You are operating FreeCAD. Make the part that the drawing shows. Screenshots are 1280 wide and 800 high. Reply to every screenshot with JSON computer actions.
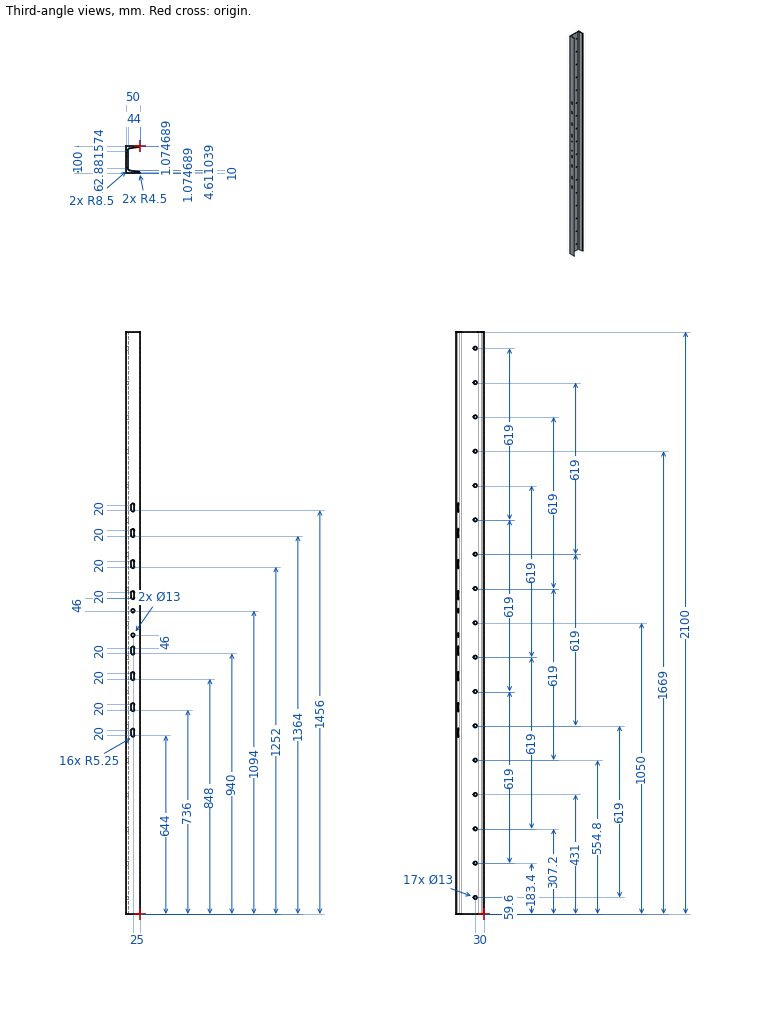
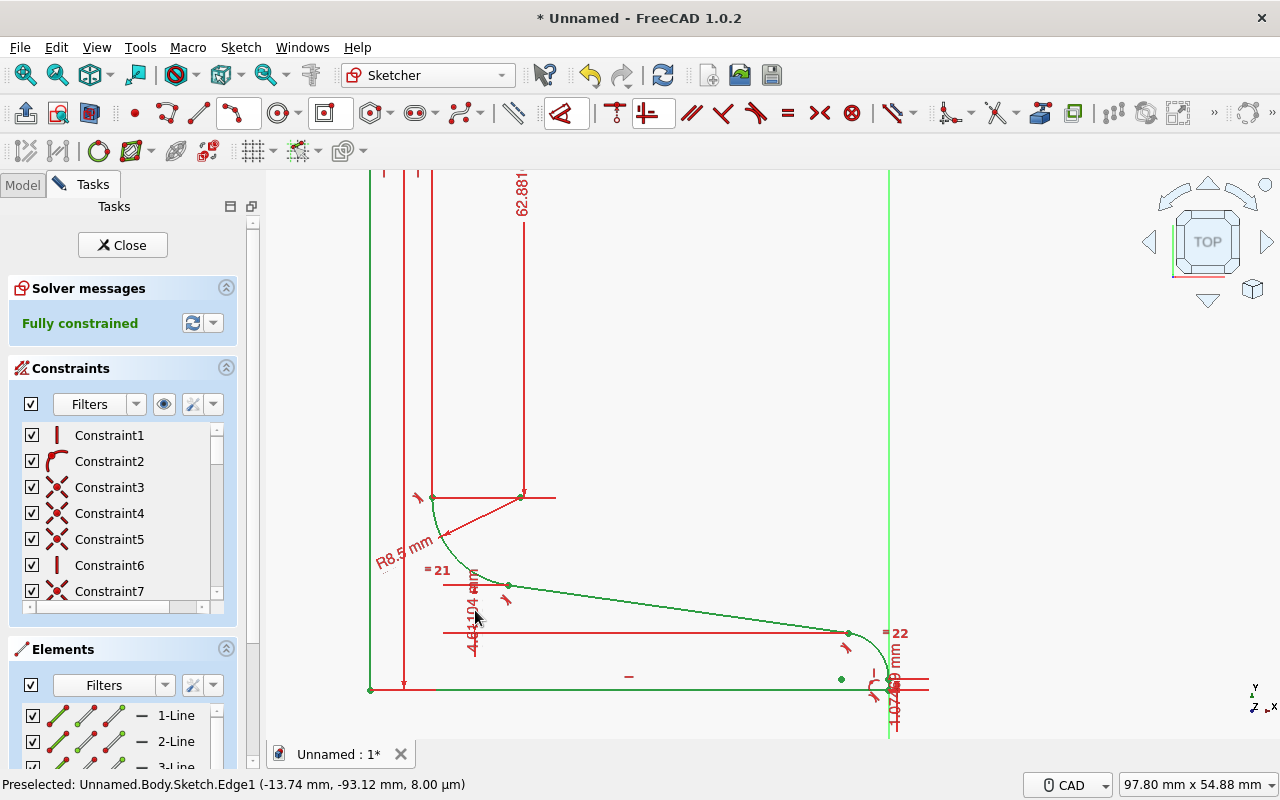
{"action": "left_click", "coordinate": [123, 245]}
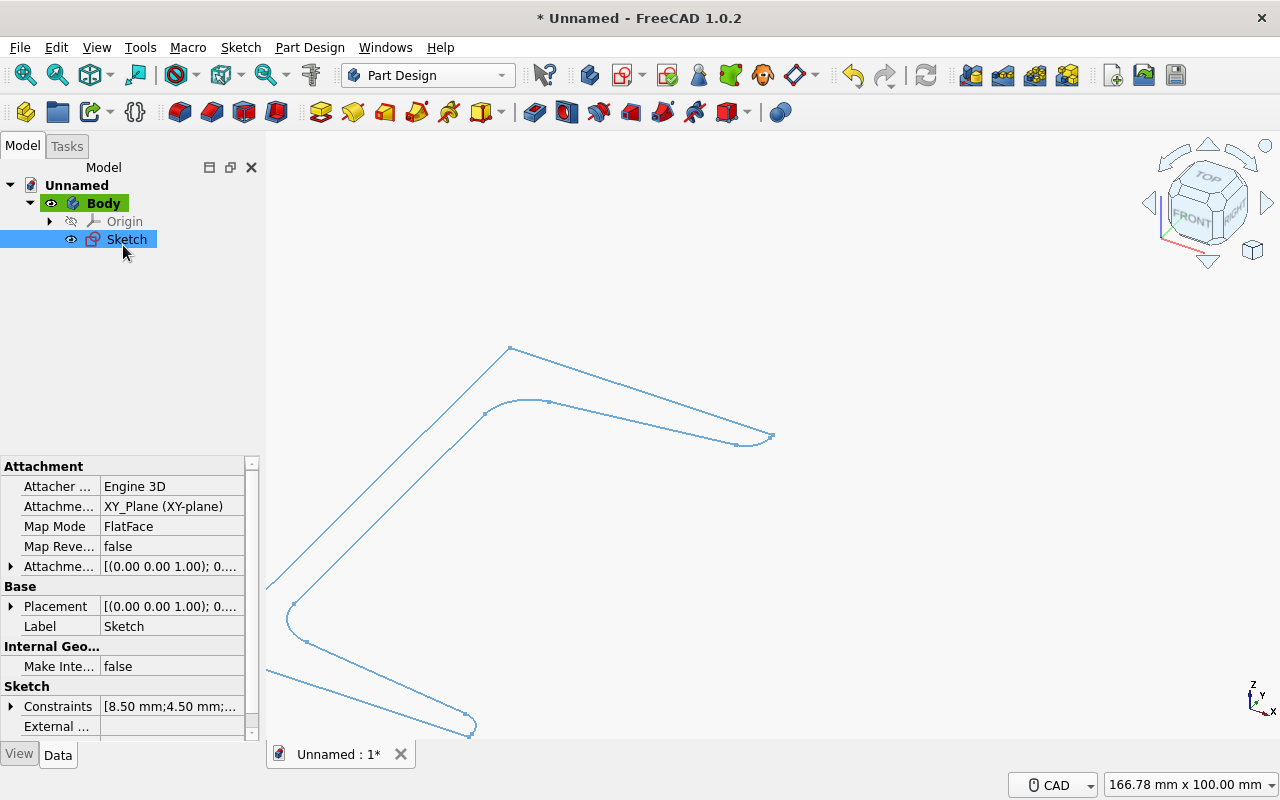
{"action": "left_click", "coordinate": [322, 112]}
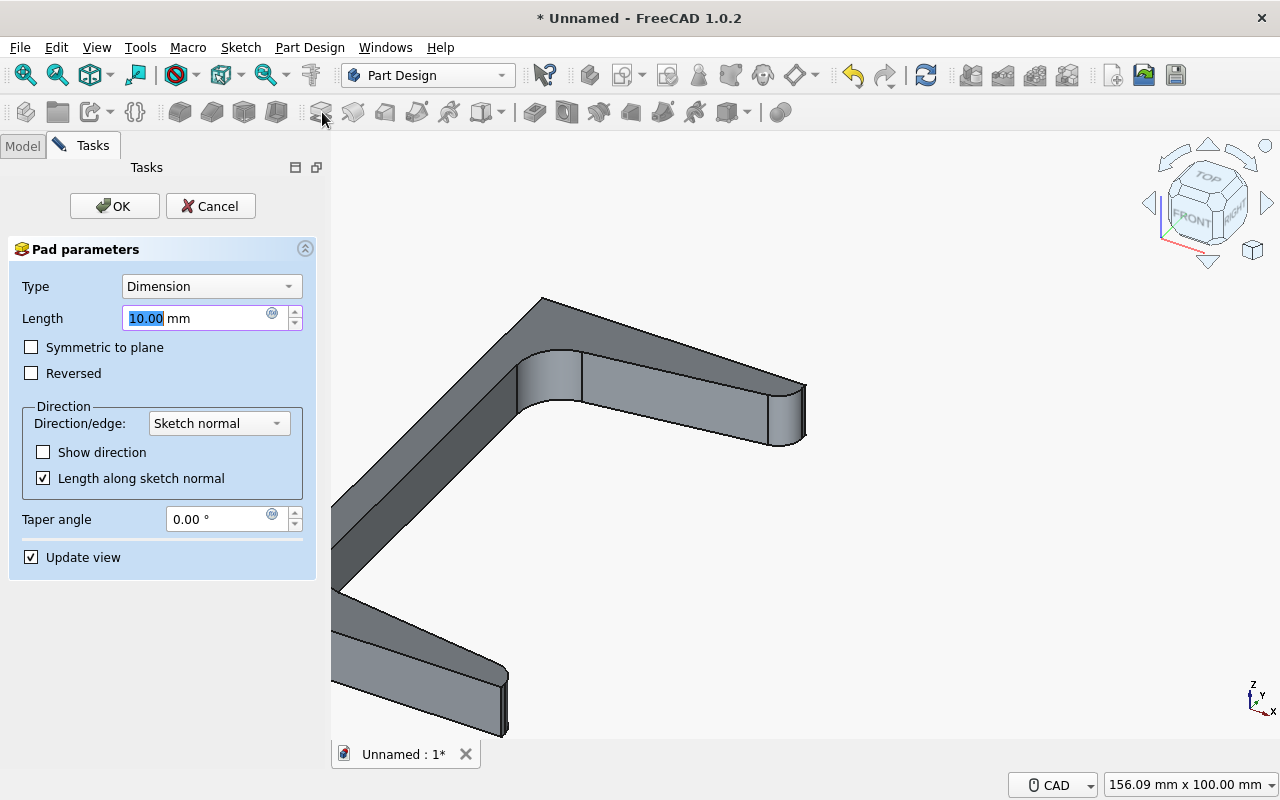
{"action": "type", "text": "2100"}
{"action": "key", "text": "Tab"}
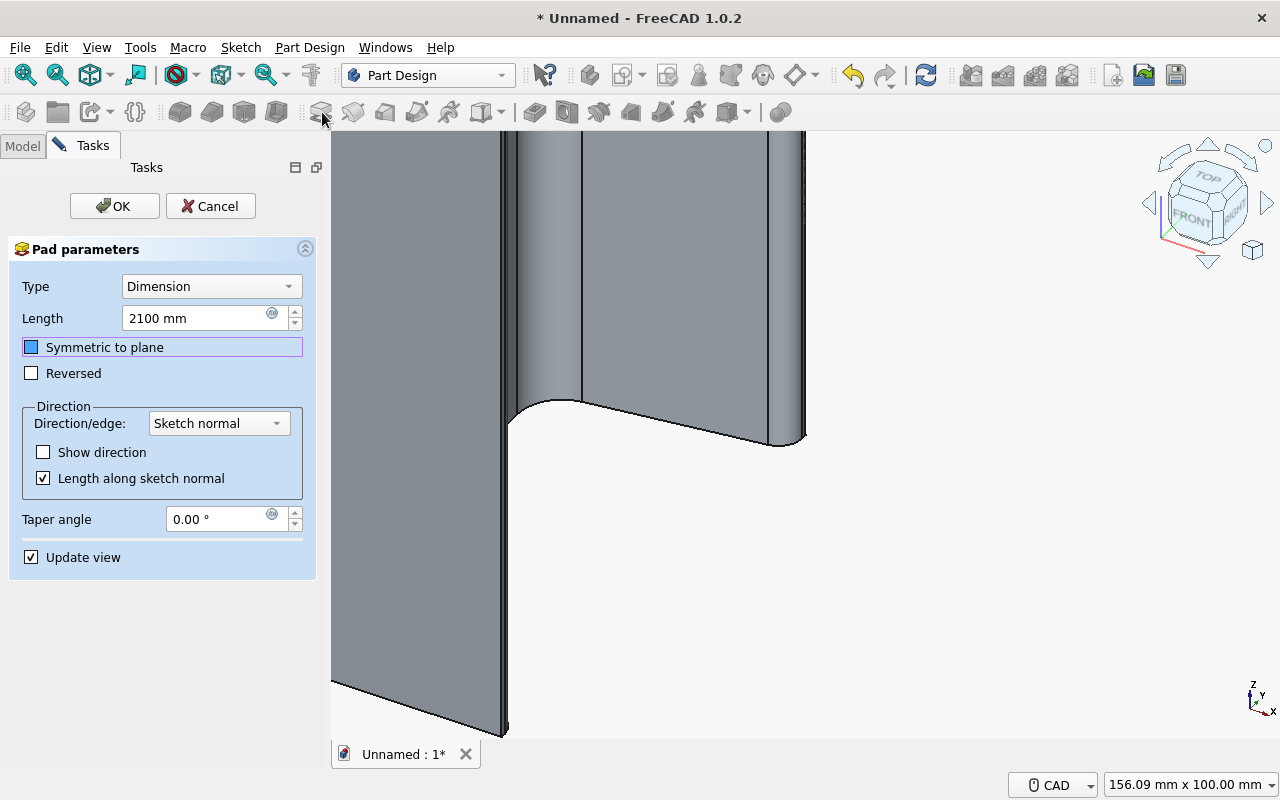
{"action": "left_click", "coordinate": [115, 206]}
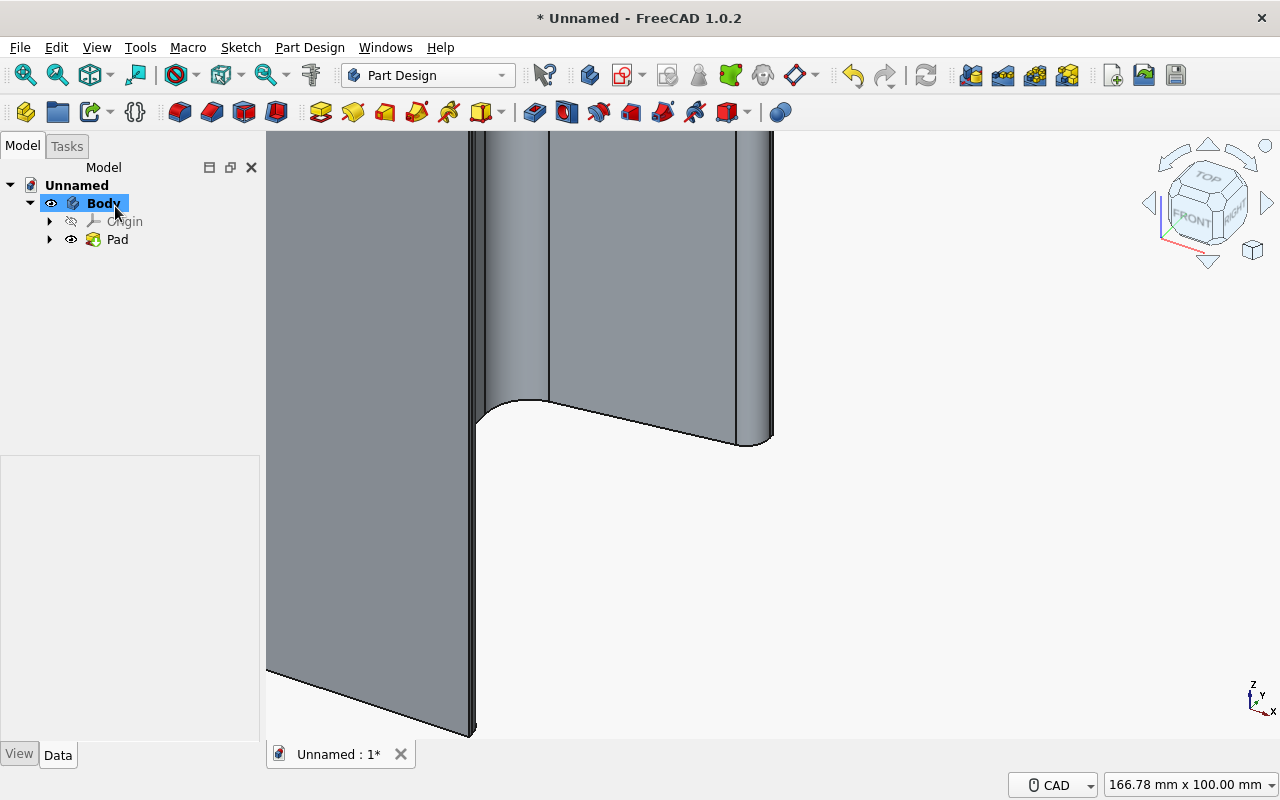
{"action": "left_click", "coordinate": [26, 76]}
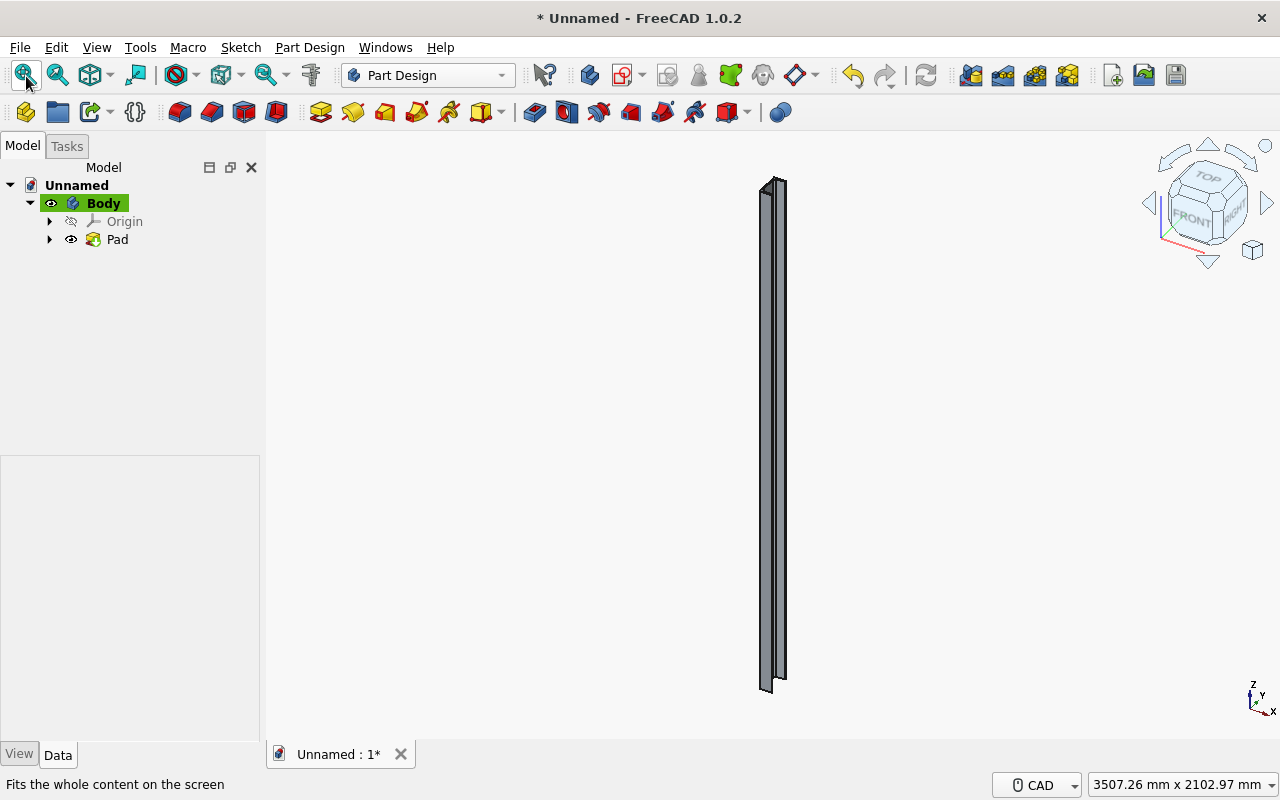
{"action": "key", "text": "6"}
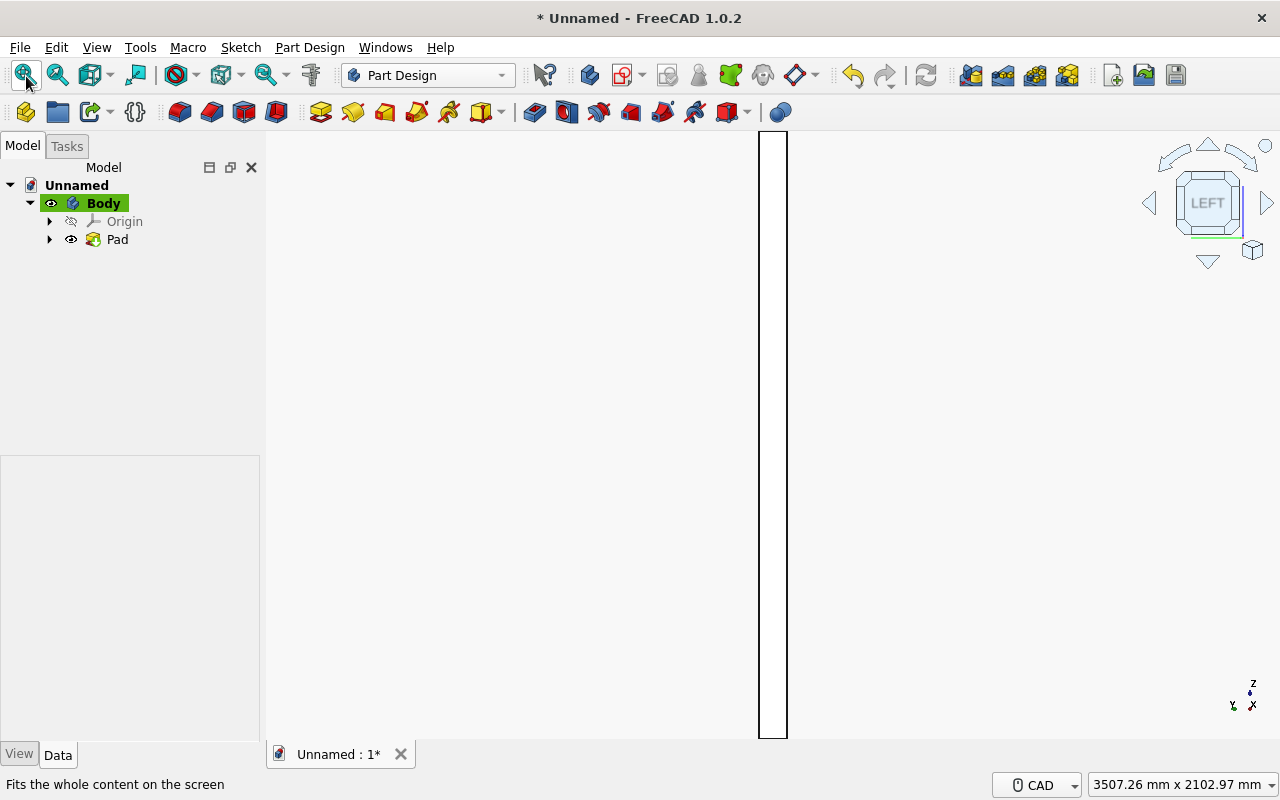
{"action": "left_click", "coordinate": [26, 76]}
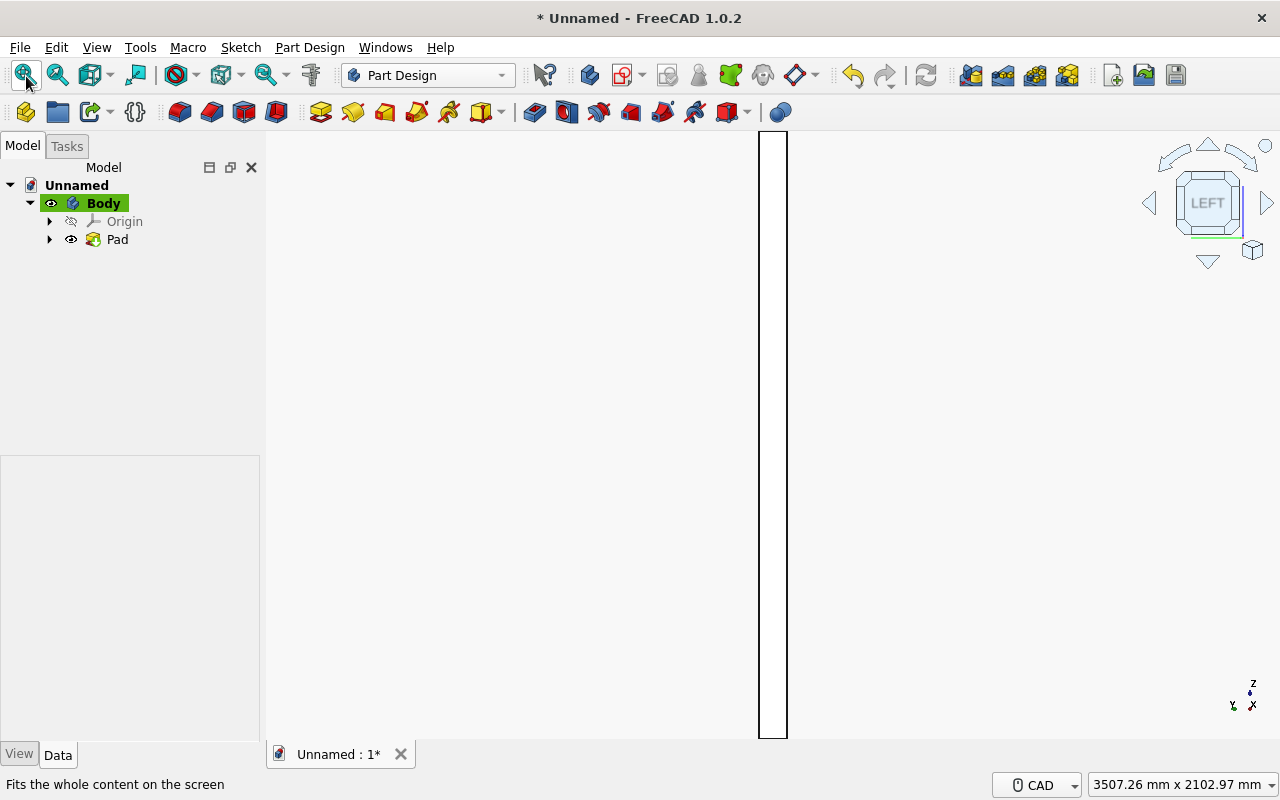
{"action": "left_click", "coordinate": [773, 174]}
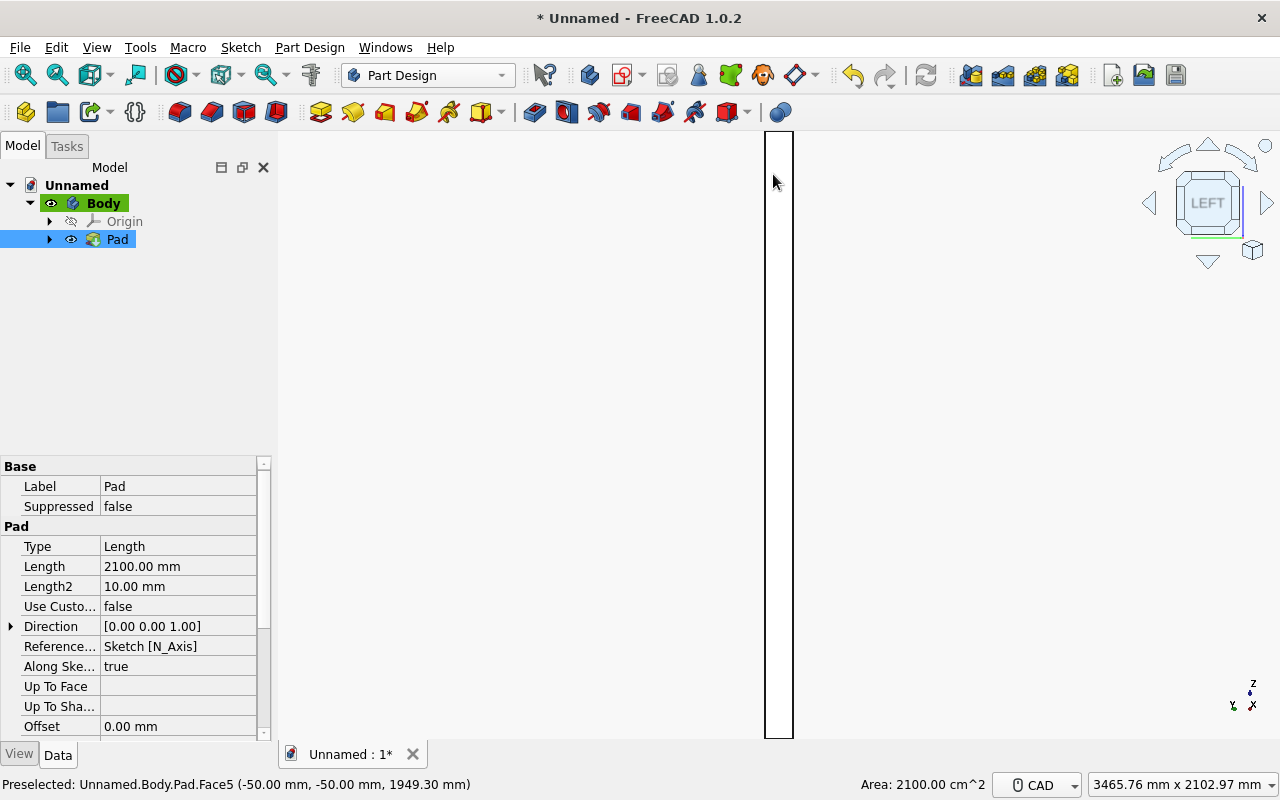
{"action": "left_click", "coordinate": [622, 76]}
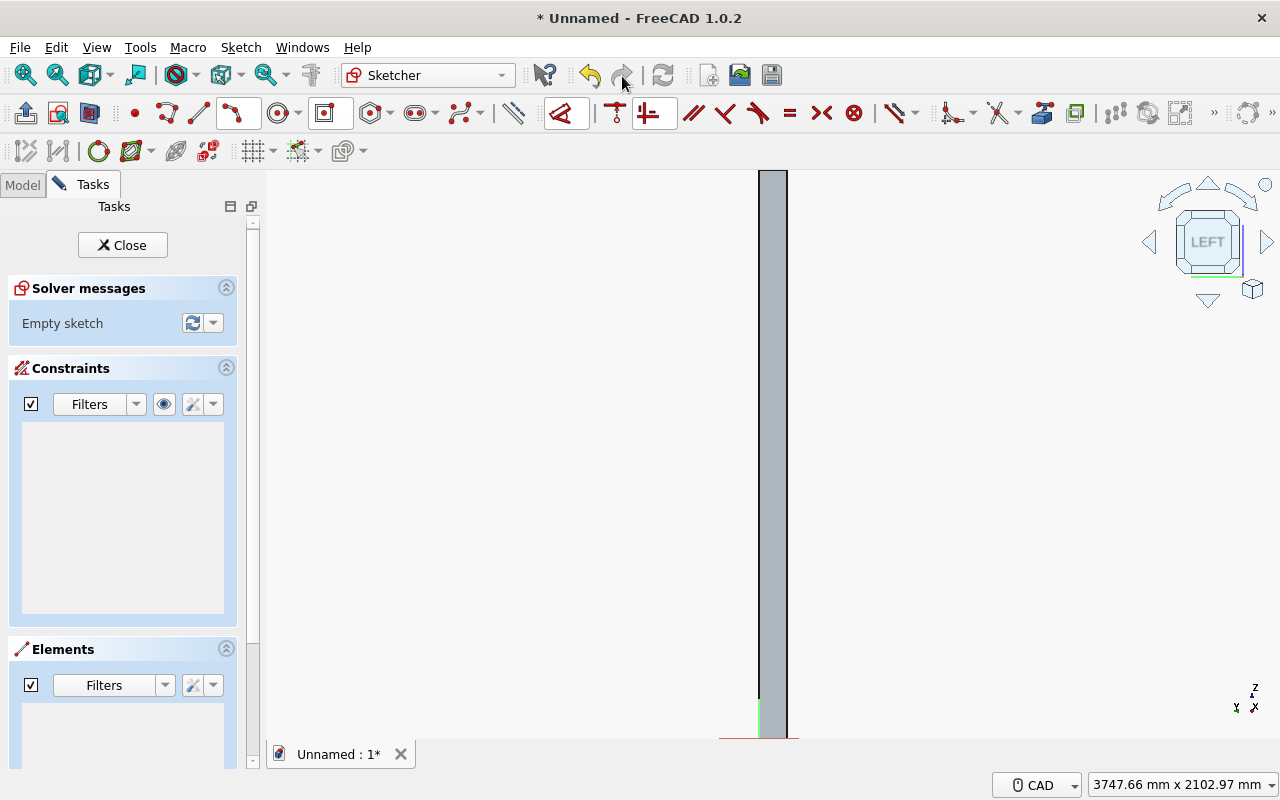
{"action": "scroll", "coordinate": [583, 440], "scroll_direction": "down", "scroll_amount": 2}